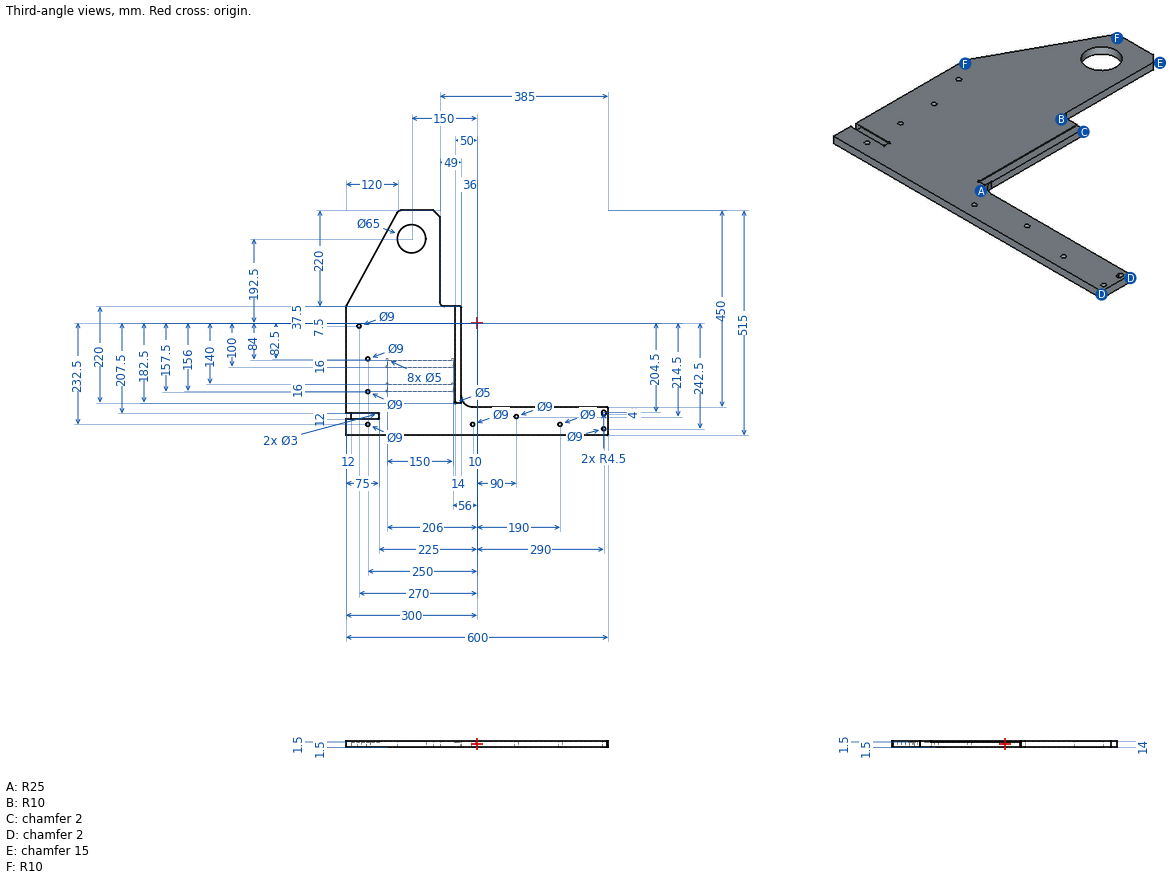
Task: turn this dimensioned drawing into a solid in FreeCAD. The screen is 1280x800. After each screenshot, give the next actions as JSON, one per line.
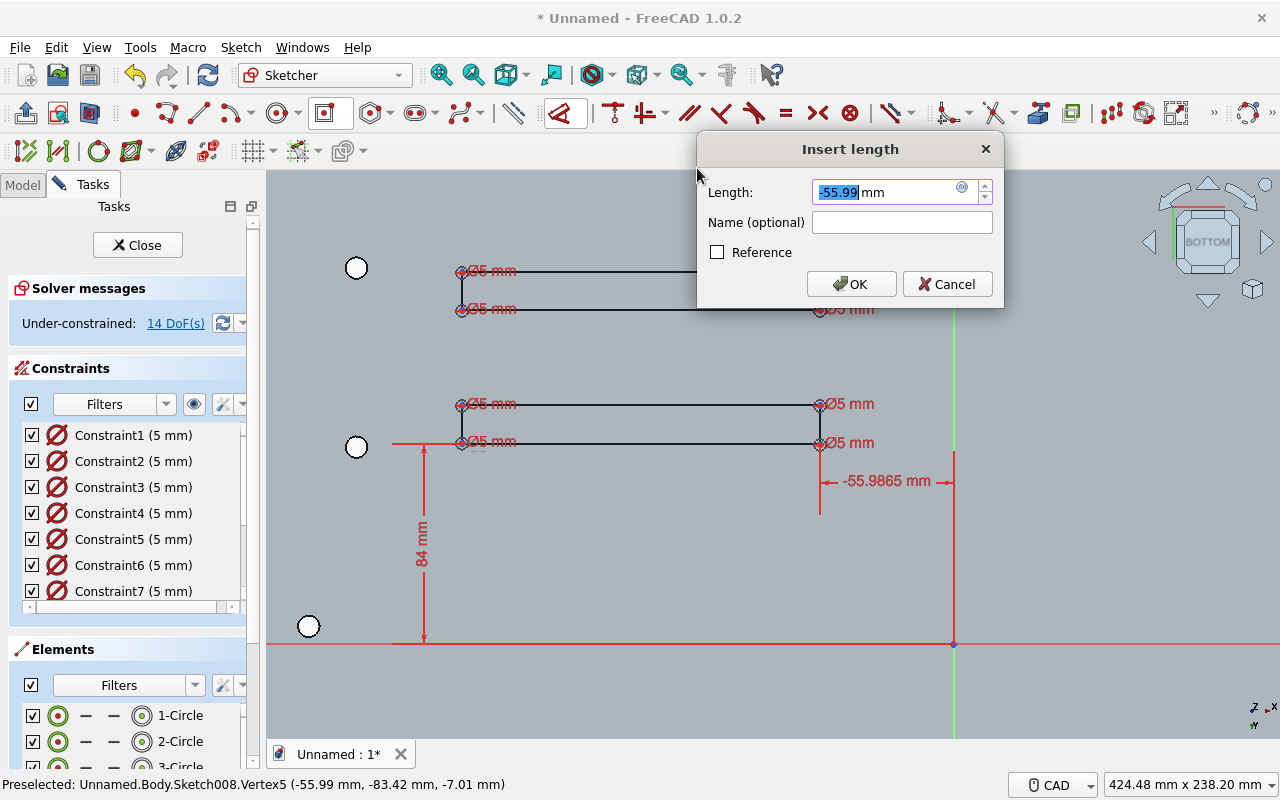
{"action": "type", "text": "-56"}
{"action": "key", "text": "Return"}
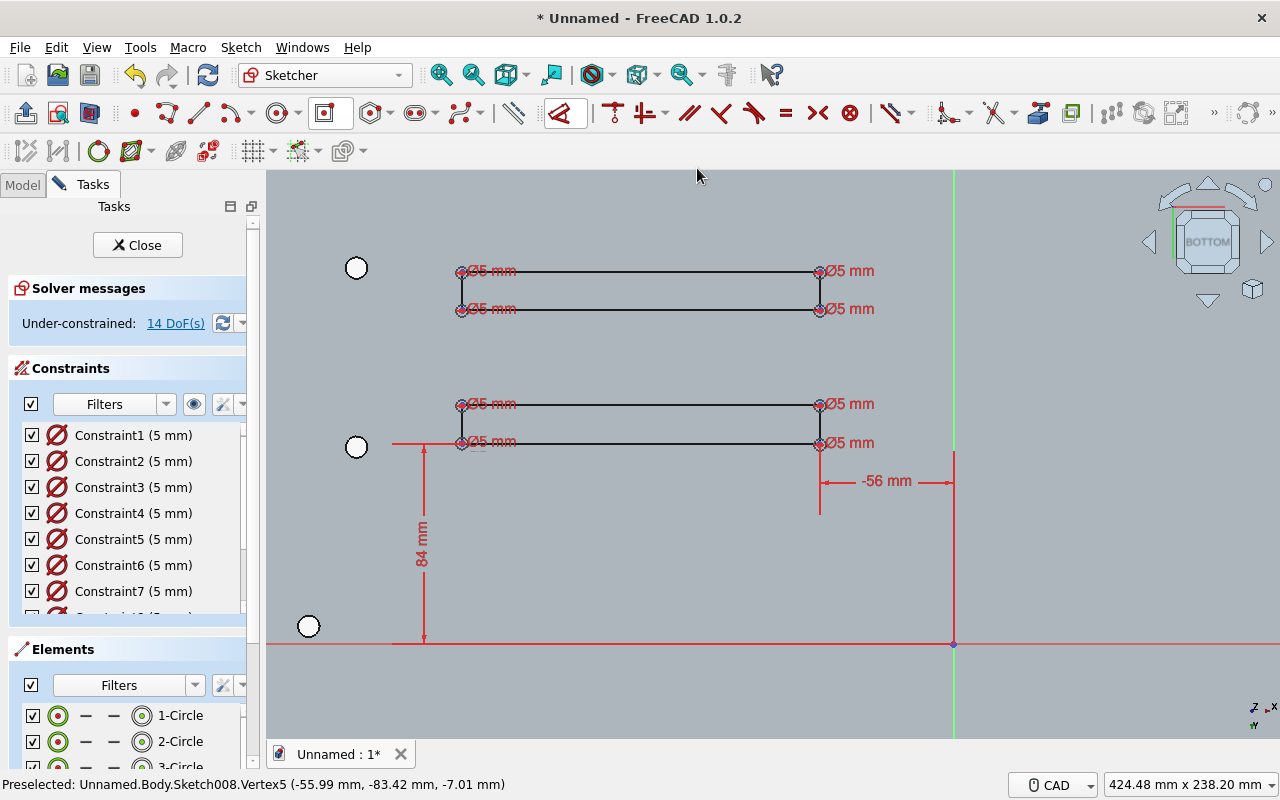
{"action": "left_click", "coordinate": [820, 445]}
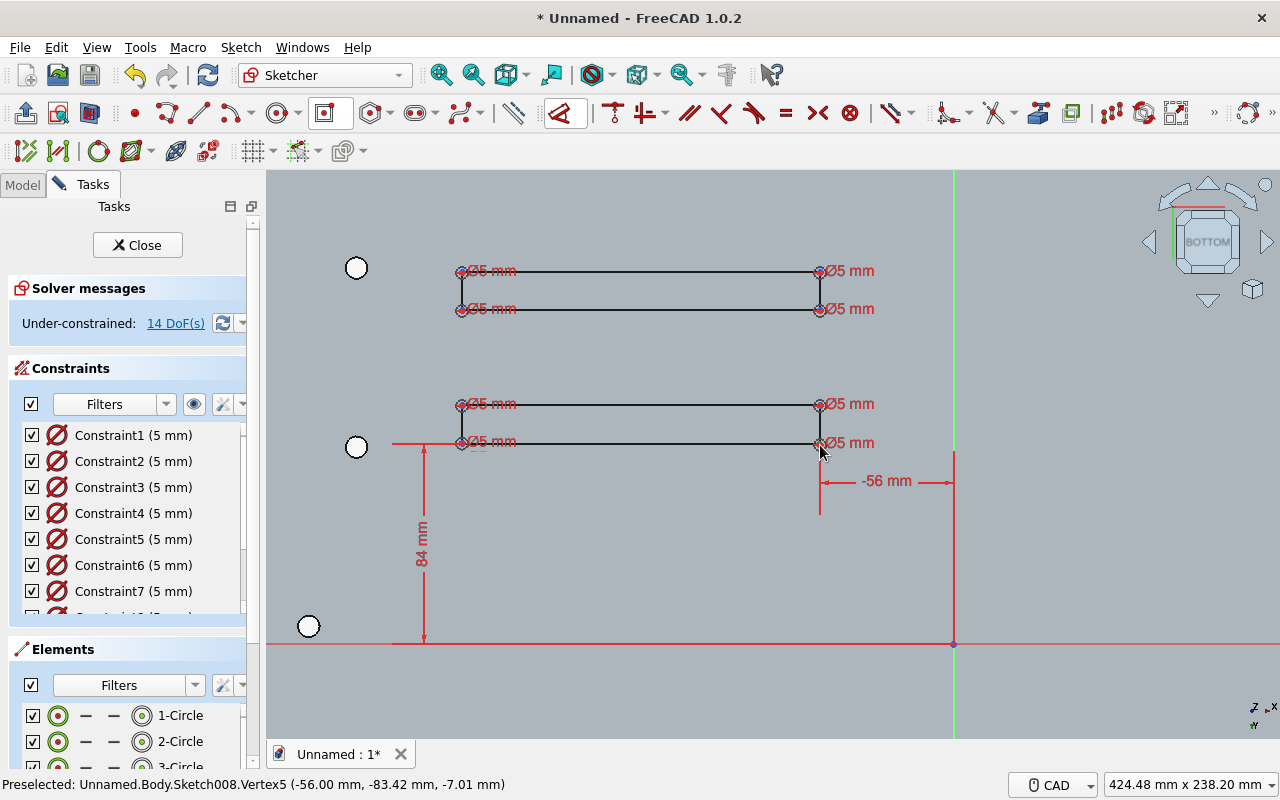
{"action": "left_click", "coordinate": [582, 114]}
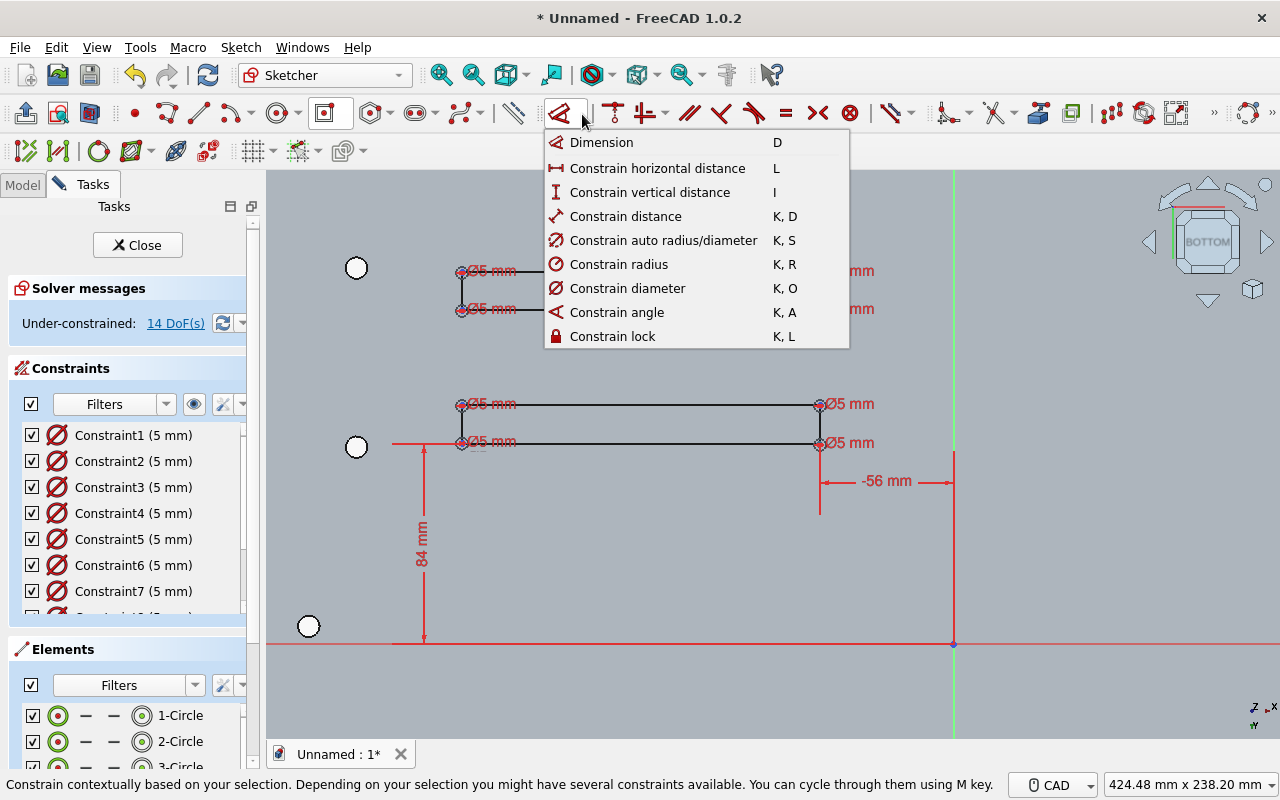
{"action": "left_click", "coordinate": [697, 192]}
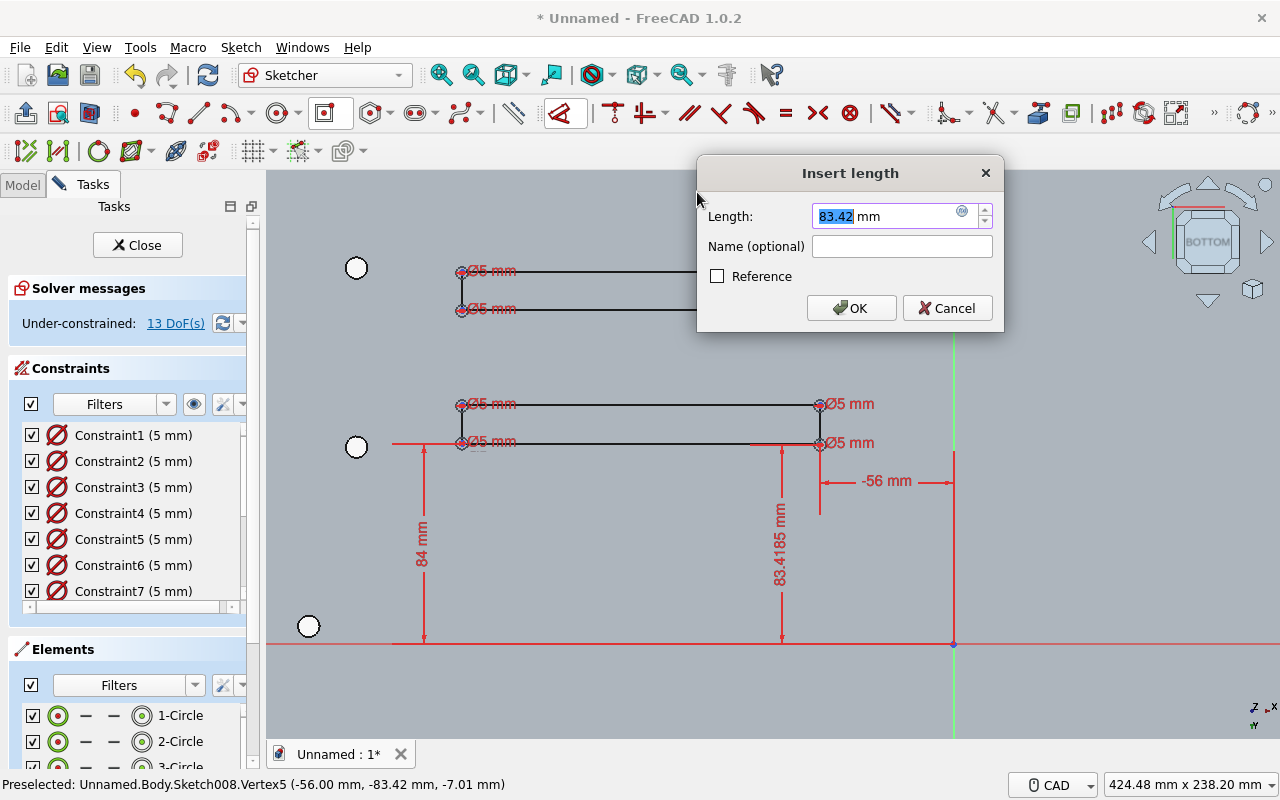
{"action": "type", "text": "84"}
{"action": "key", "text": "Return"}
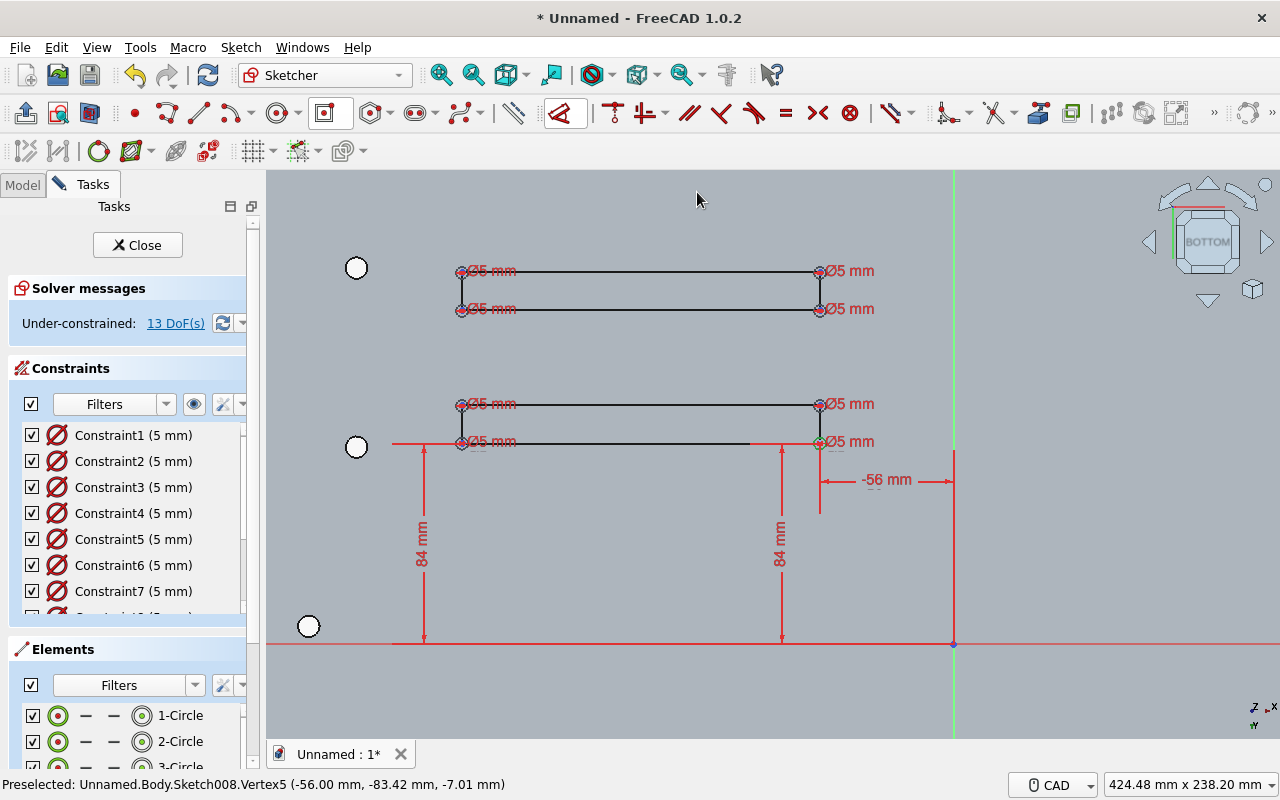
{"action": "left_click", "coordinate": [820, 406]}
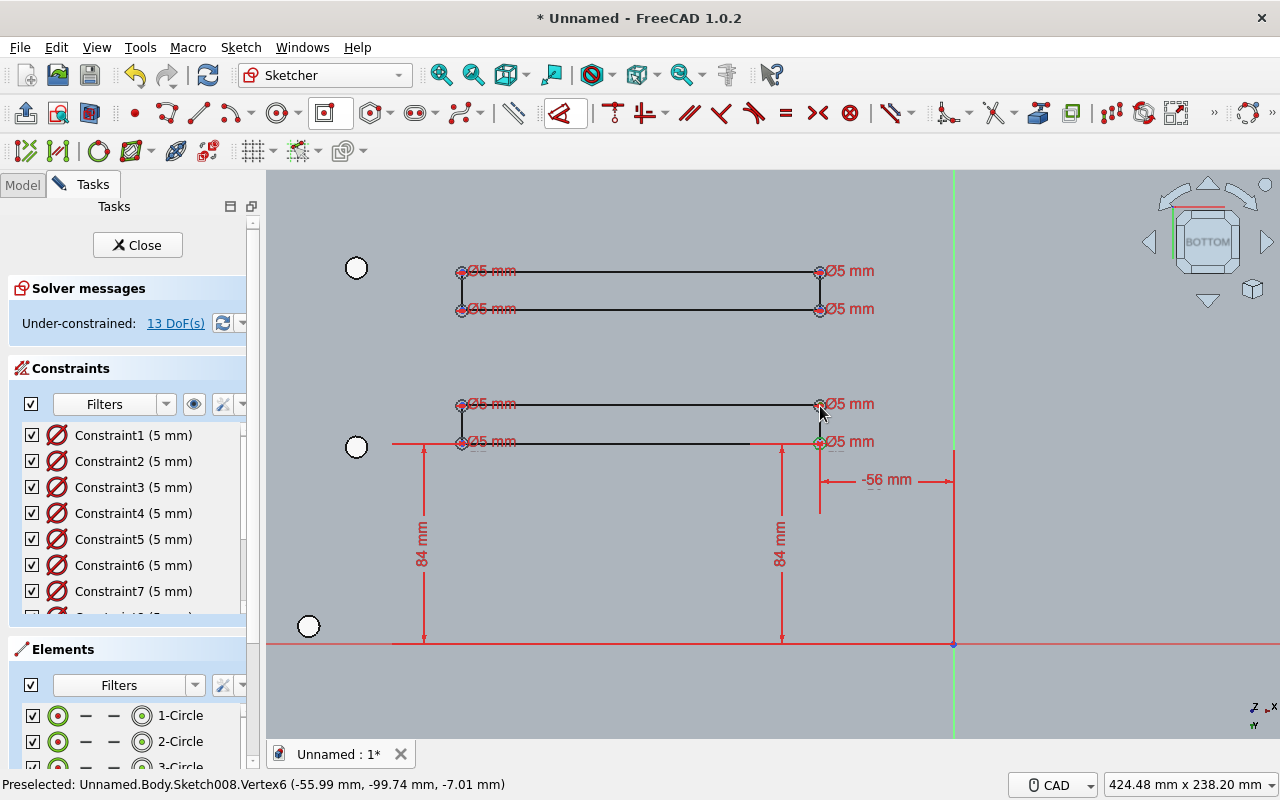
{"action": "left_click", "coordinate": [582, 114]}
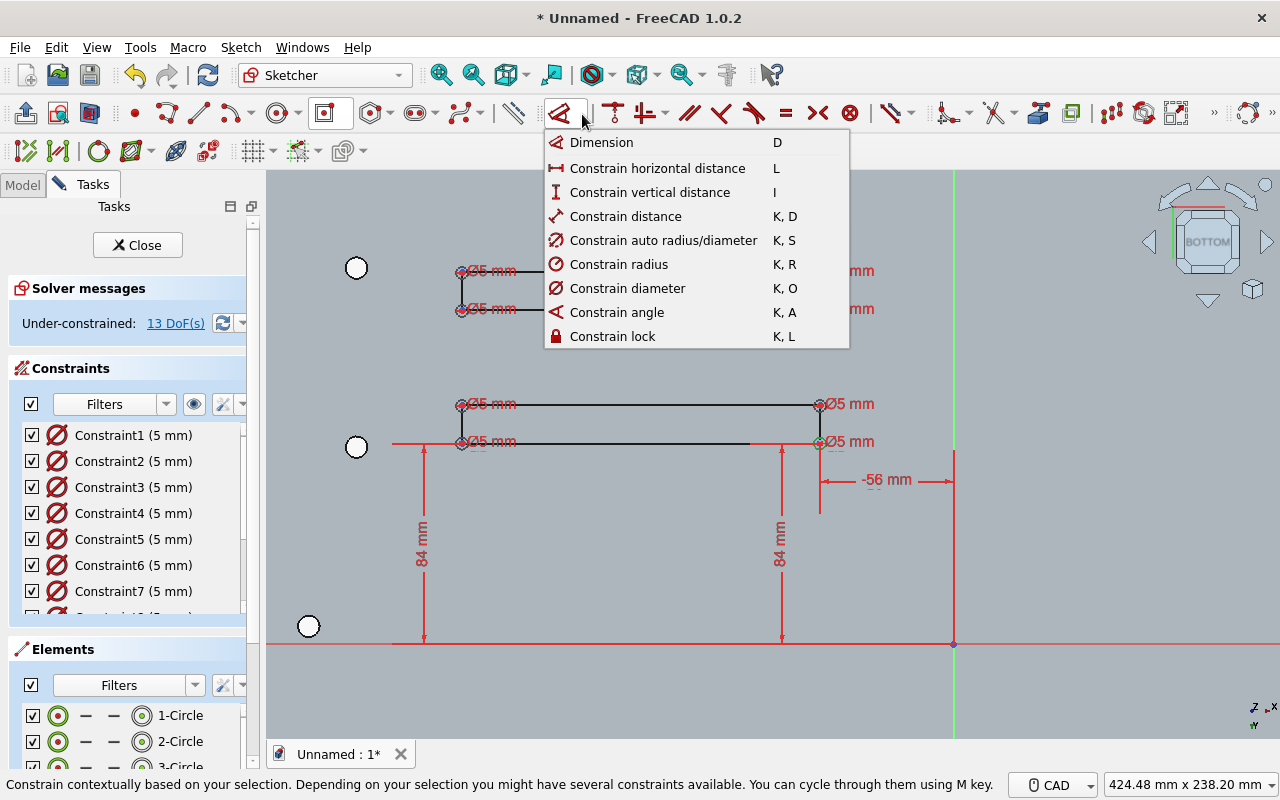
{"action": "left_click", "coordinate": [697, 168]}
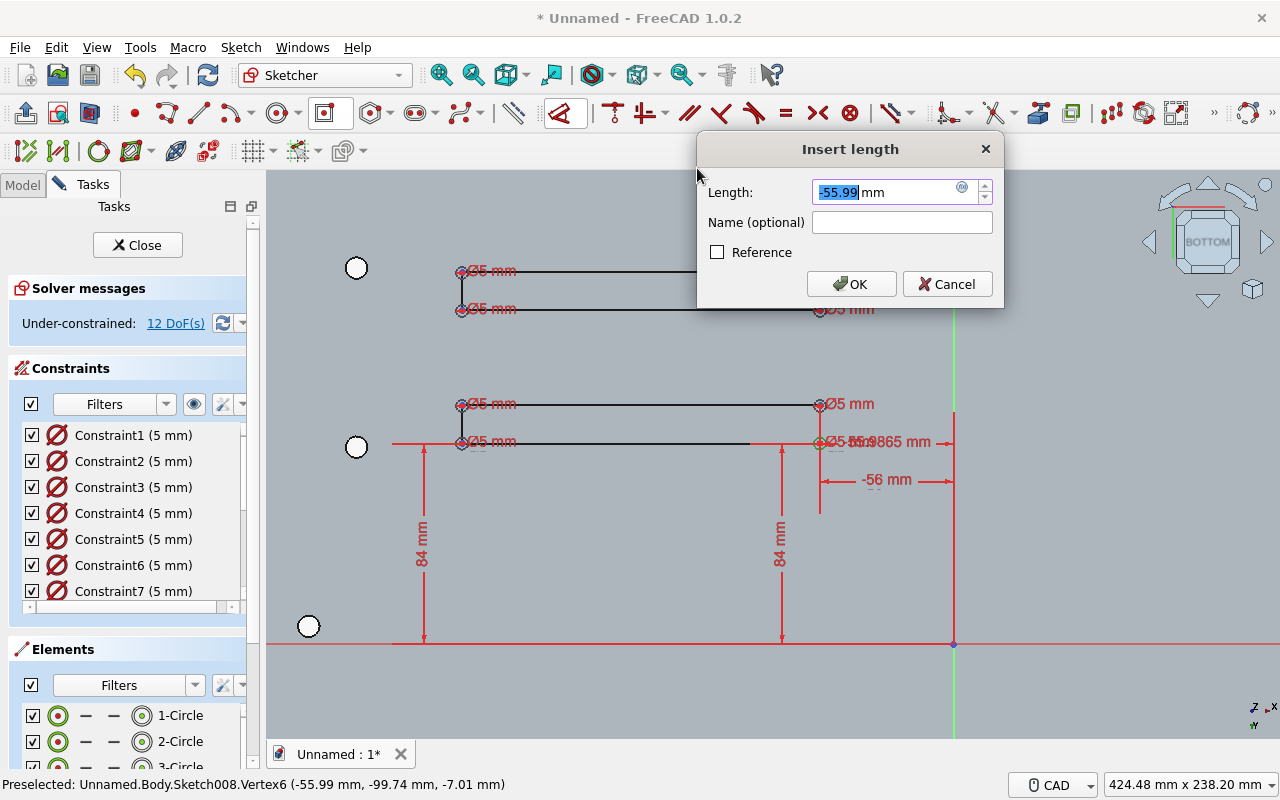
{"action": "type", "text": "-56"}
{"action": "key", "text": "Return"}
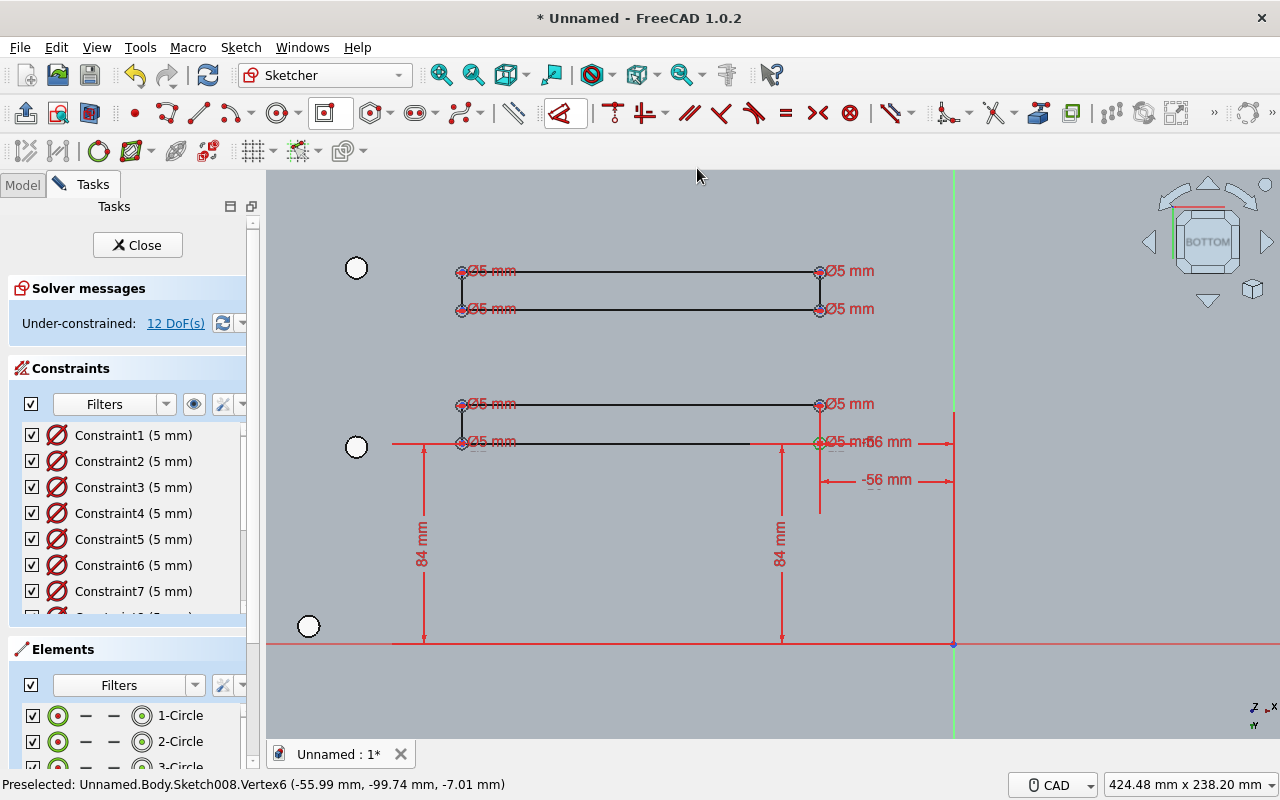
{"action": "left_click", "coordinate": [820, 311]}